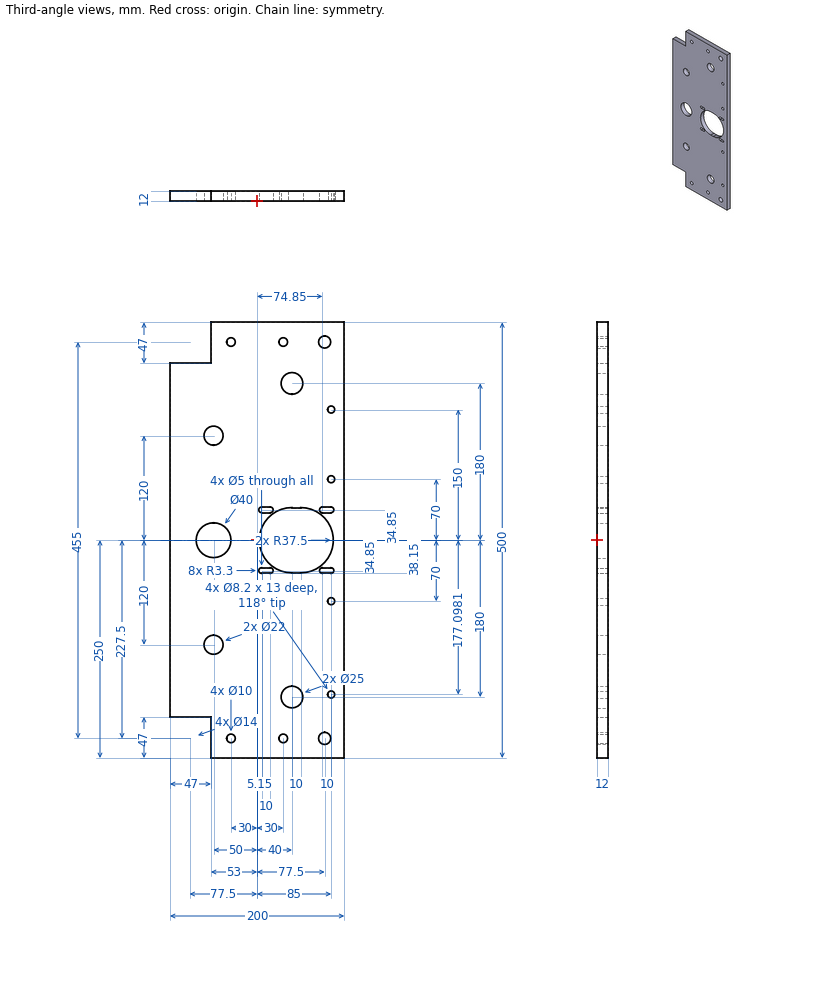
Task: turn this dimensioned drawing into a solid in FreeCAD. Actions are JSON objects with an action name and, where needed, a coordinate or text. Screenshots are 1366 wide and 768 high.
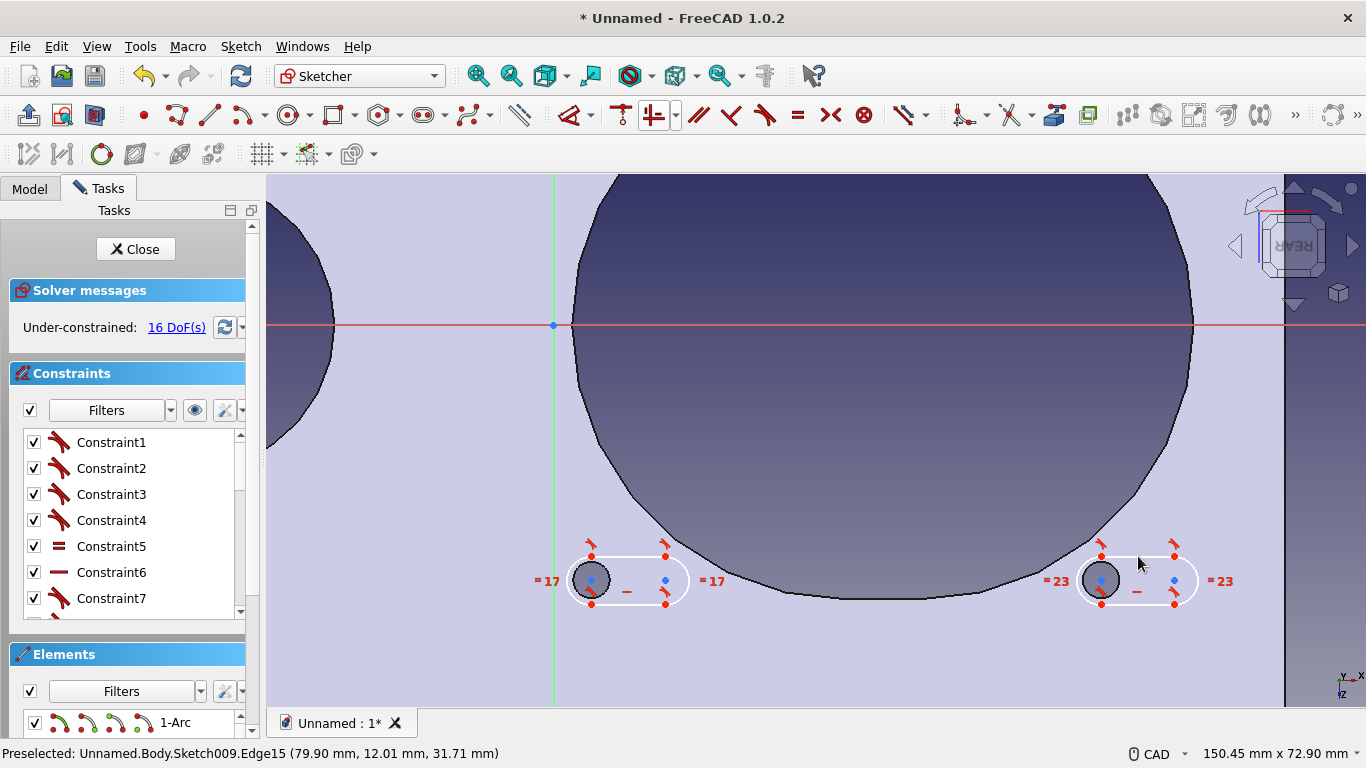
{"action": "scroll", "coordinate": [591, 581], "scroll_direction": "down", "scroll_amount": 3}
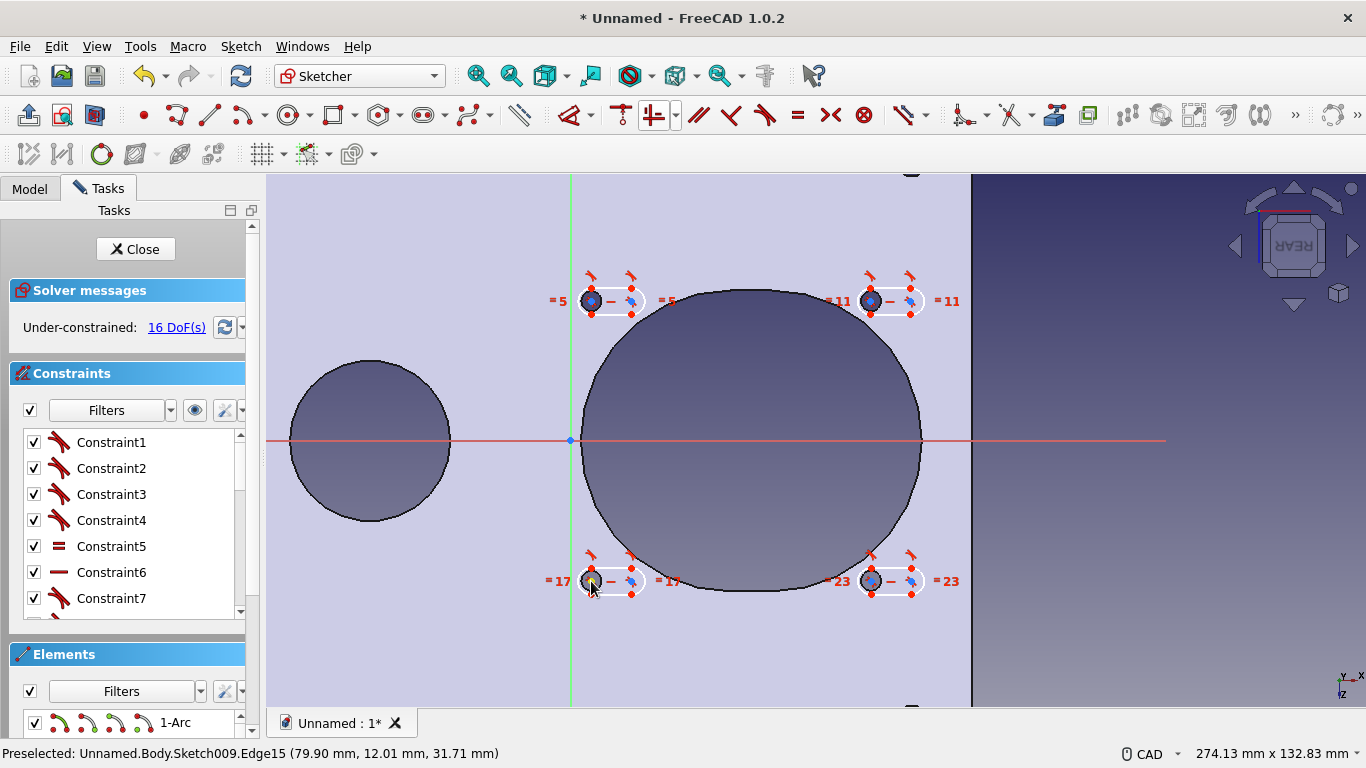
{"action": "scroll", "coordinate": [581, 294], "scroll_direction": "up", "scroll_amount": 2}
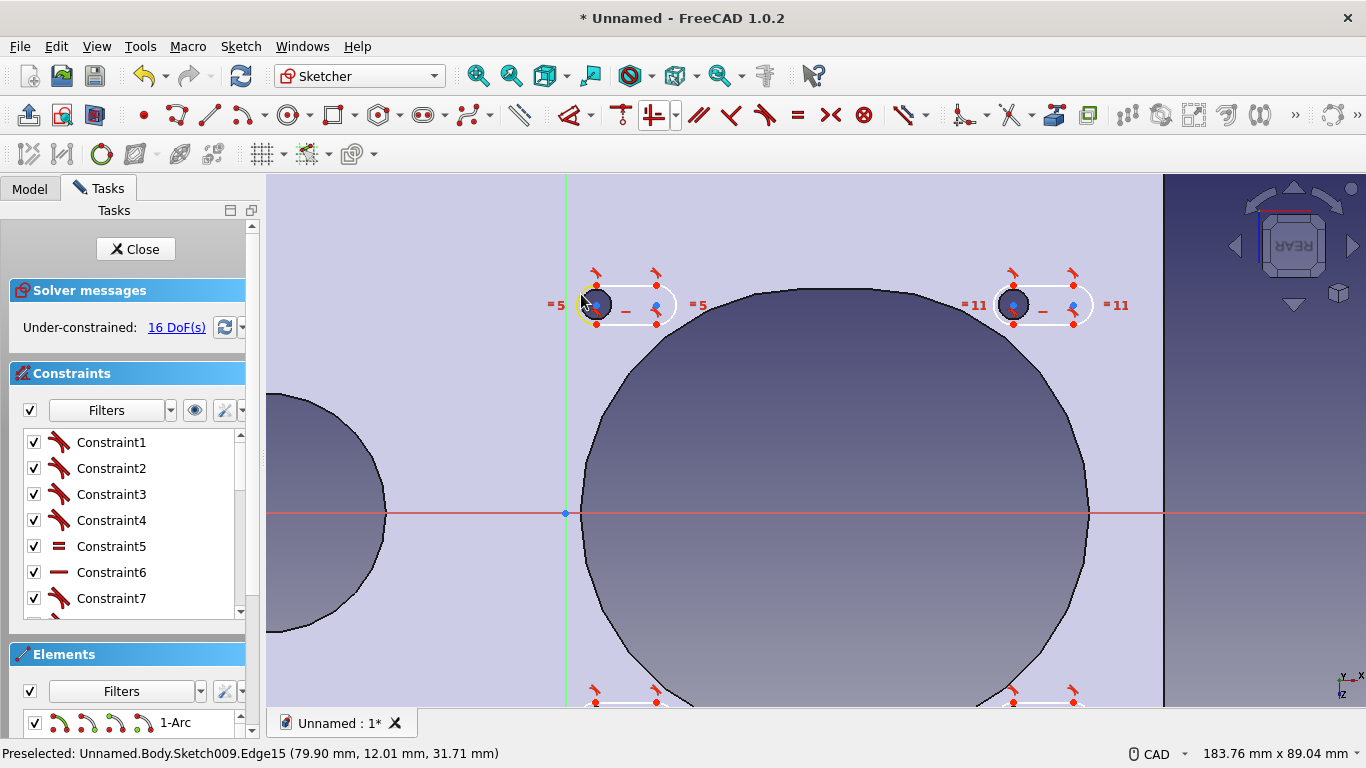
{"action": "left_click", "coordinate": [581, 294]}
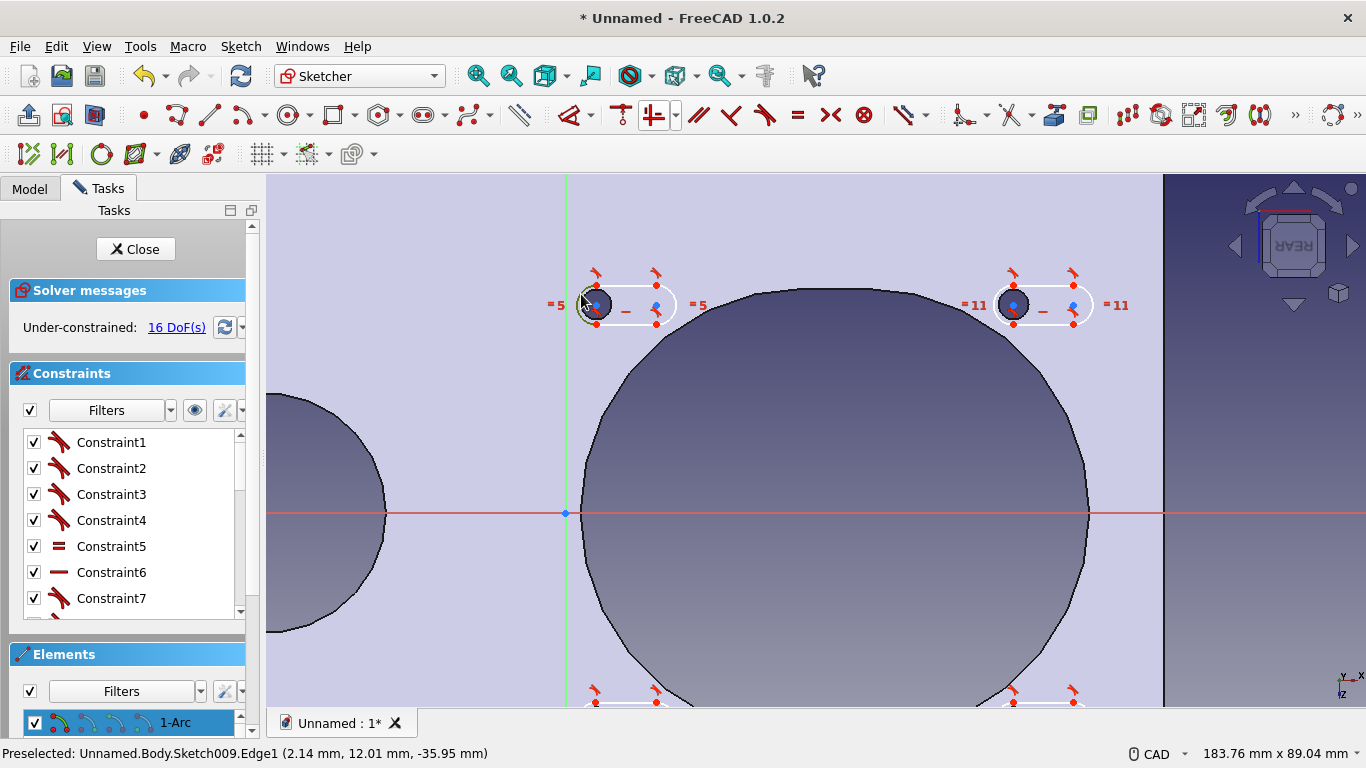
{"action": "left_click", "coordinate": [997, 294]}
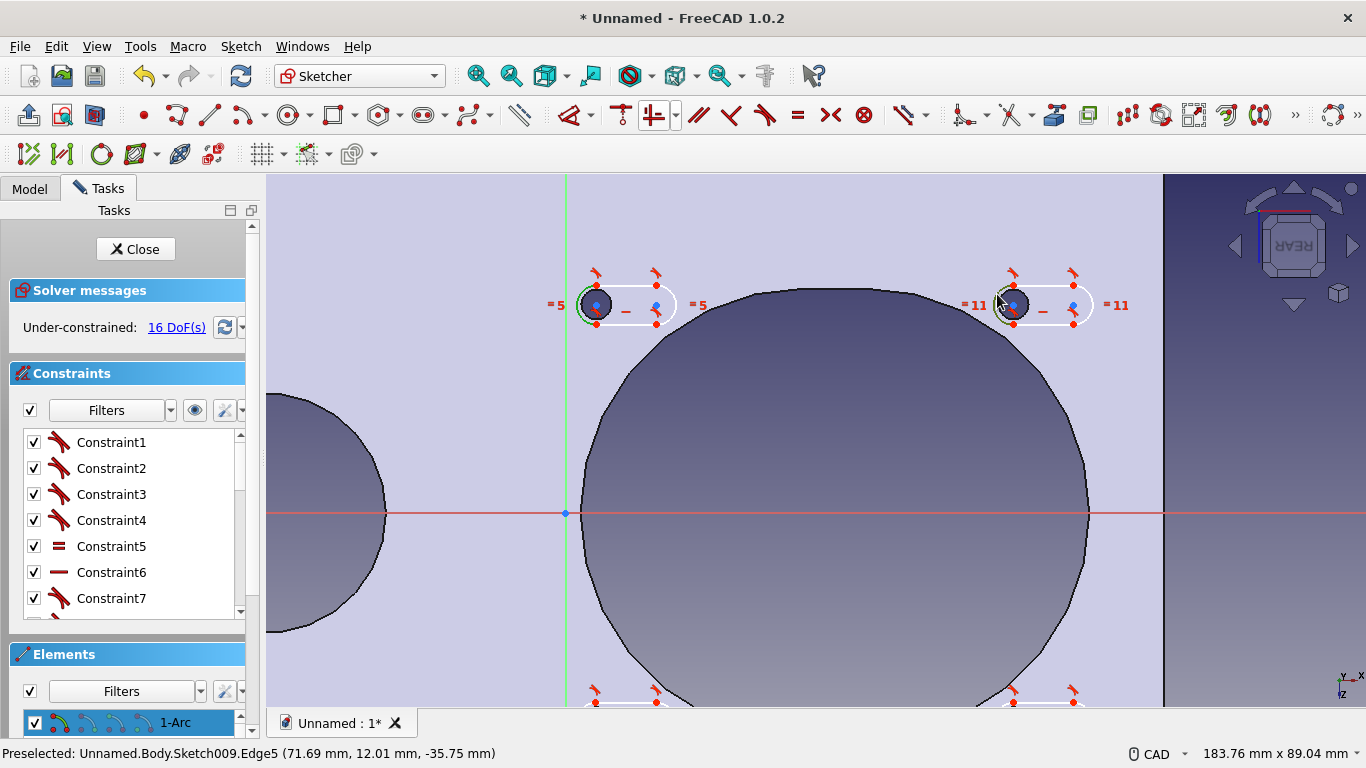
{"action": "scroll", "coordinate": [581, 293], "scroll_direction": "down", "scroll_amount": 2}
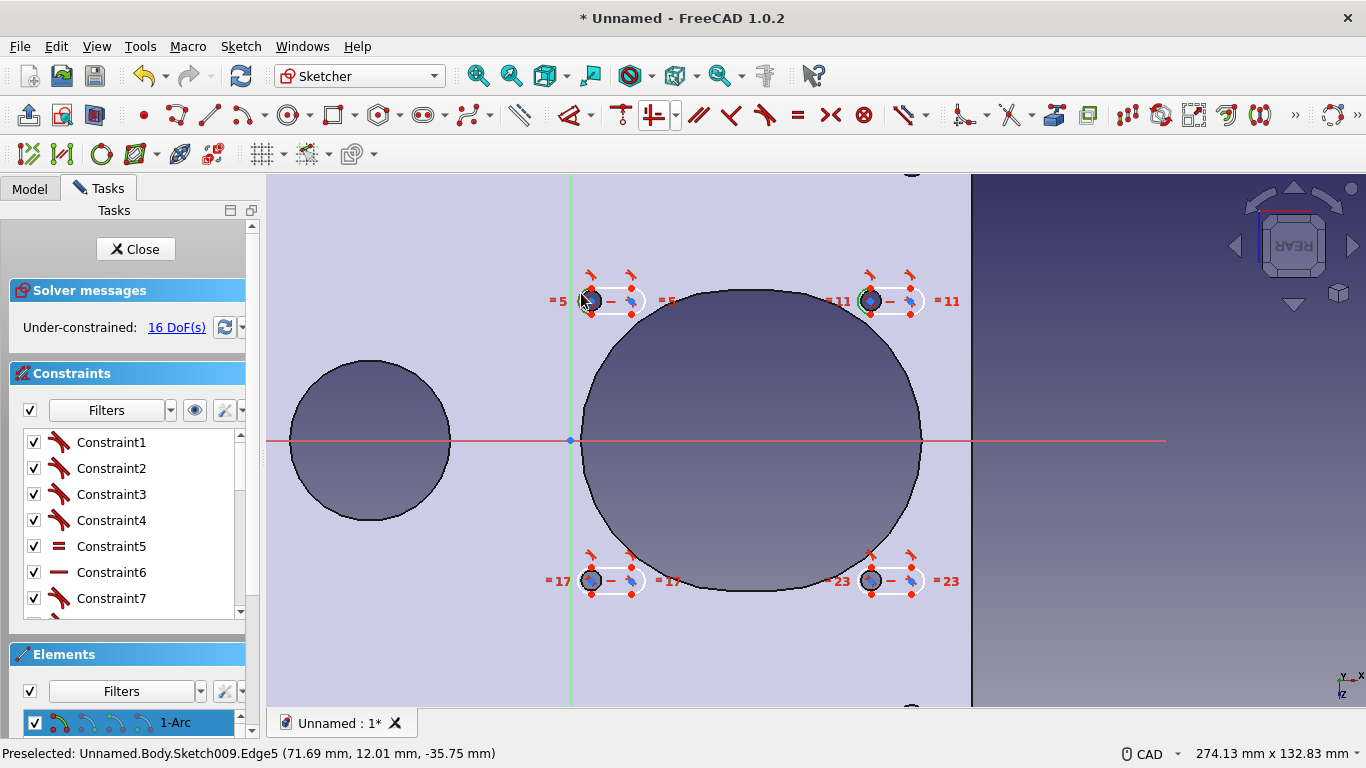
{"action": "scroll", "coordinate": [580, 573], "scroll_direction": "up", "scroll_amount": 2}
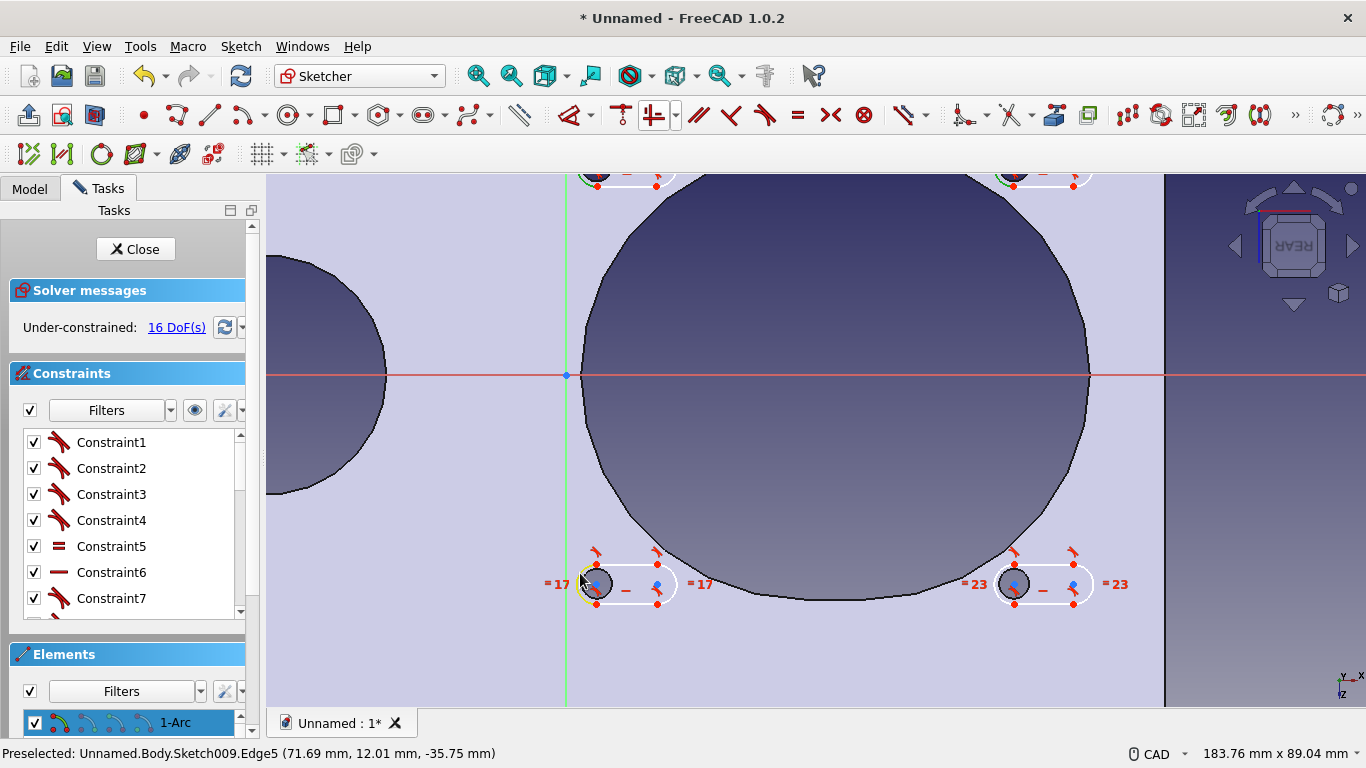
{"action": "left_click", "coordinate": [581, 573]}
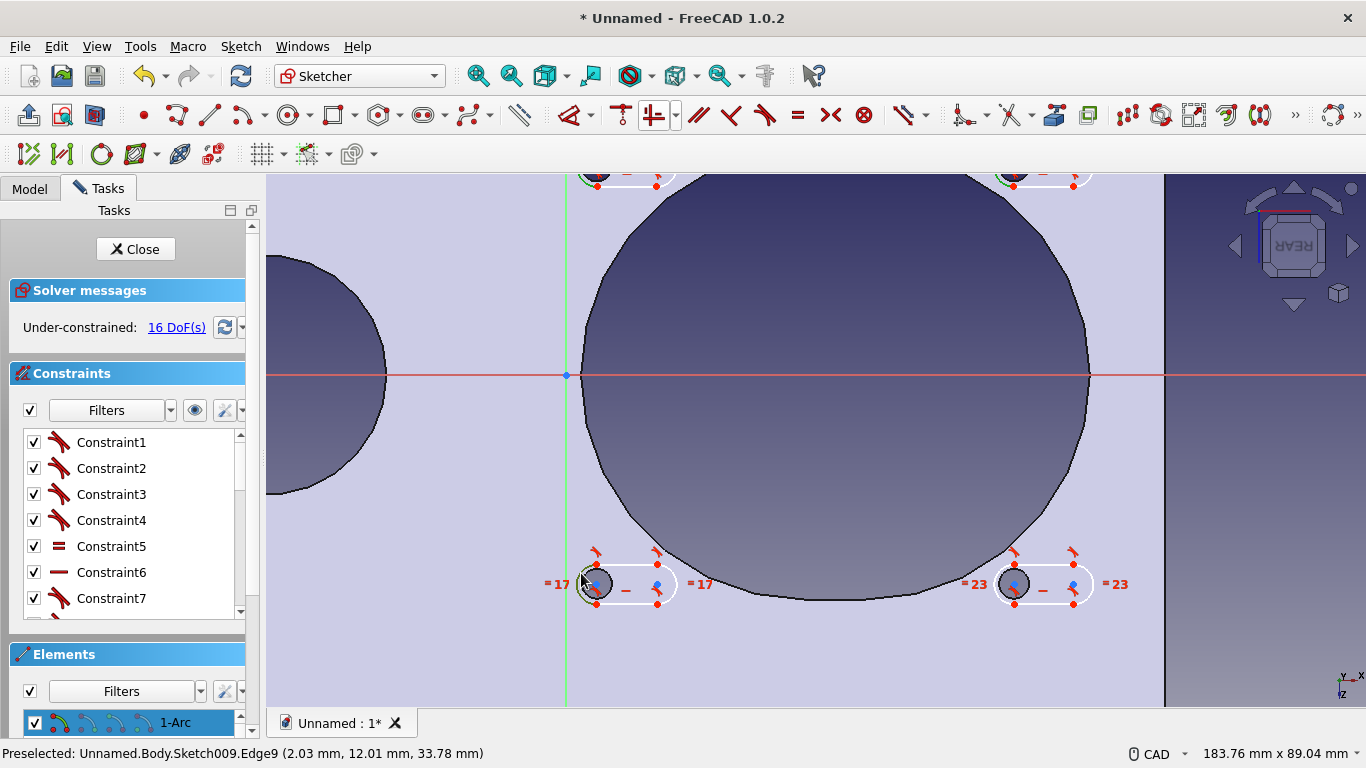
{"action": "left_click", "coordinate": [998, 573]}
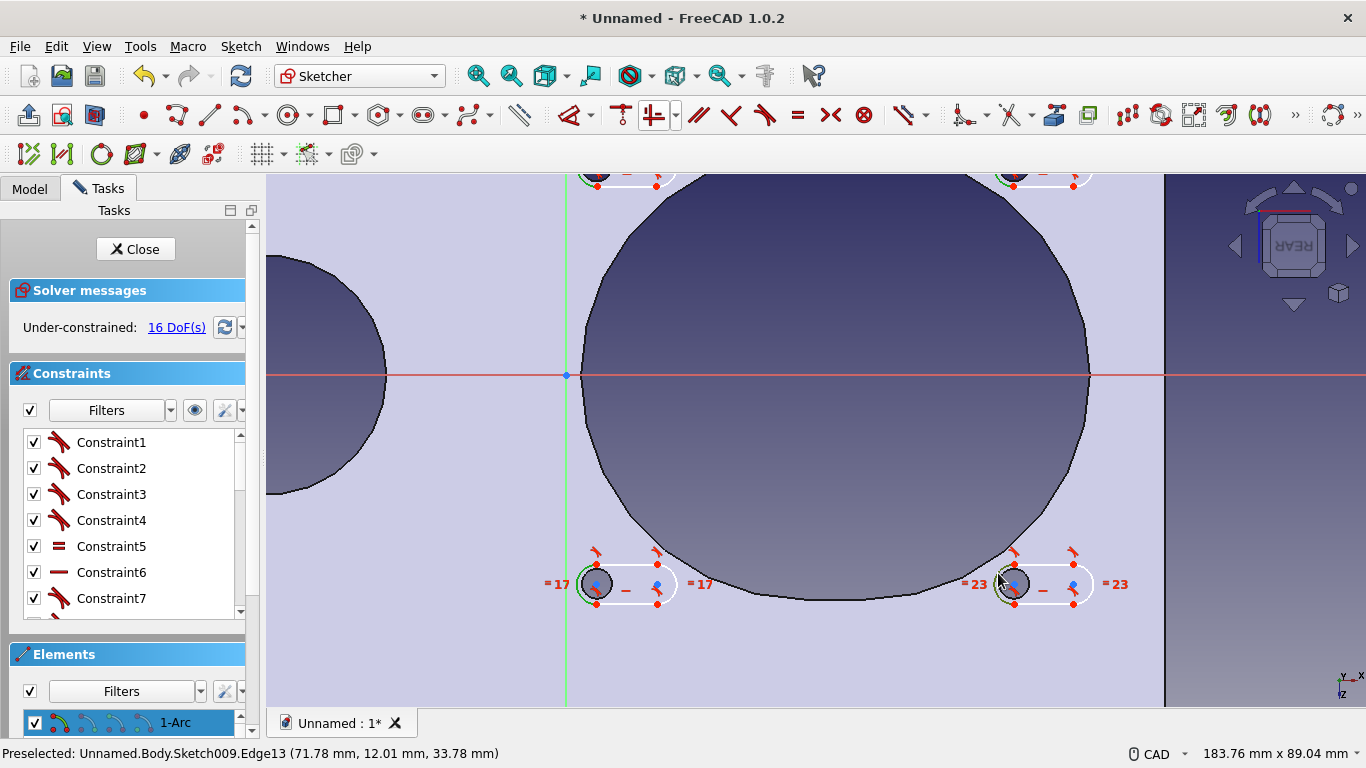
{"action": "left_click", "coordinate": [798, 116]}